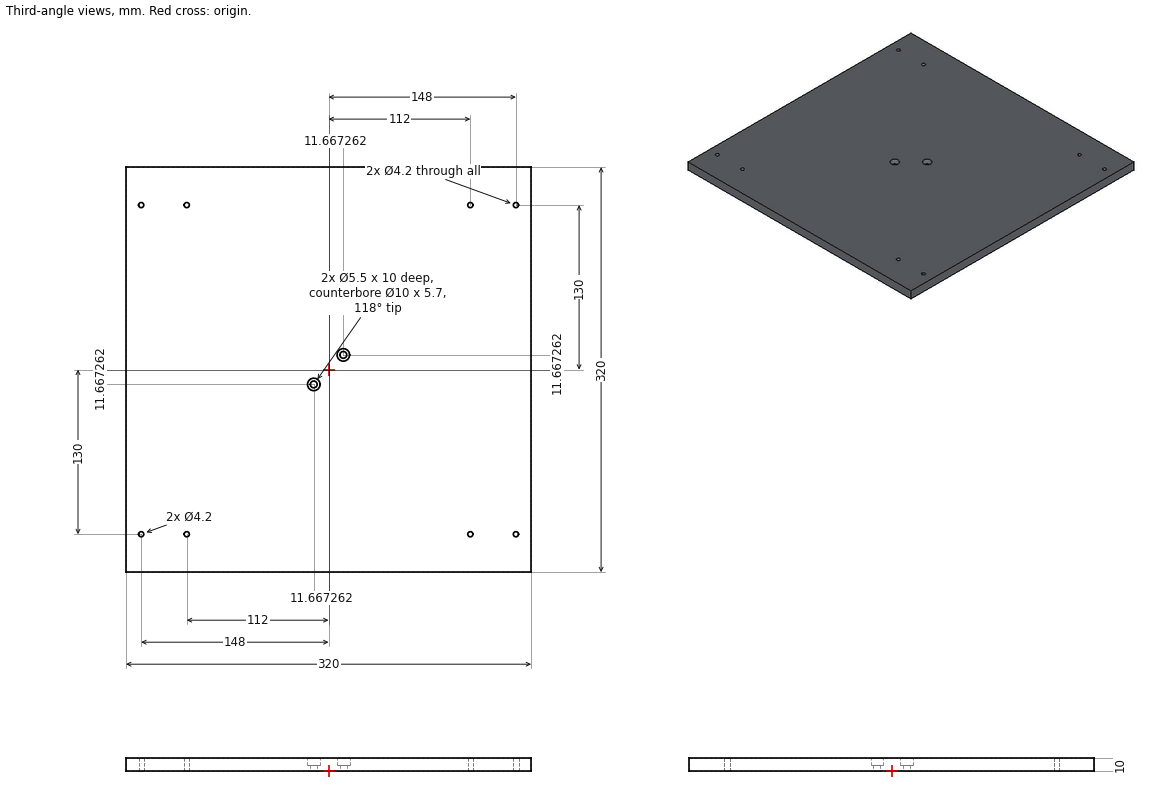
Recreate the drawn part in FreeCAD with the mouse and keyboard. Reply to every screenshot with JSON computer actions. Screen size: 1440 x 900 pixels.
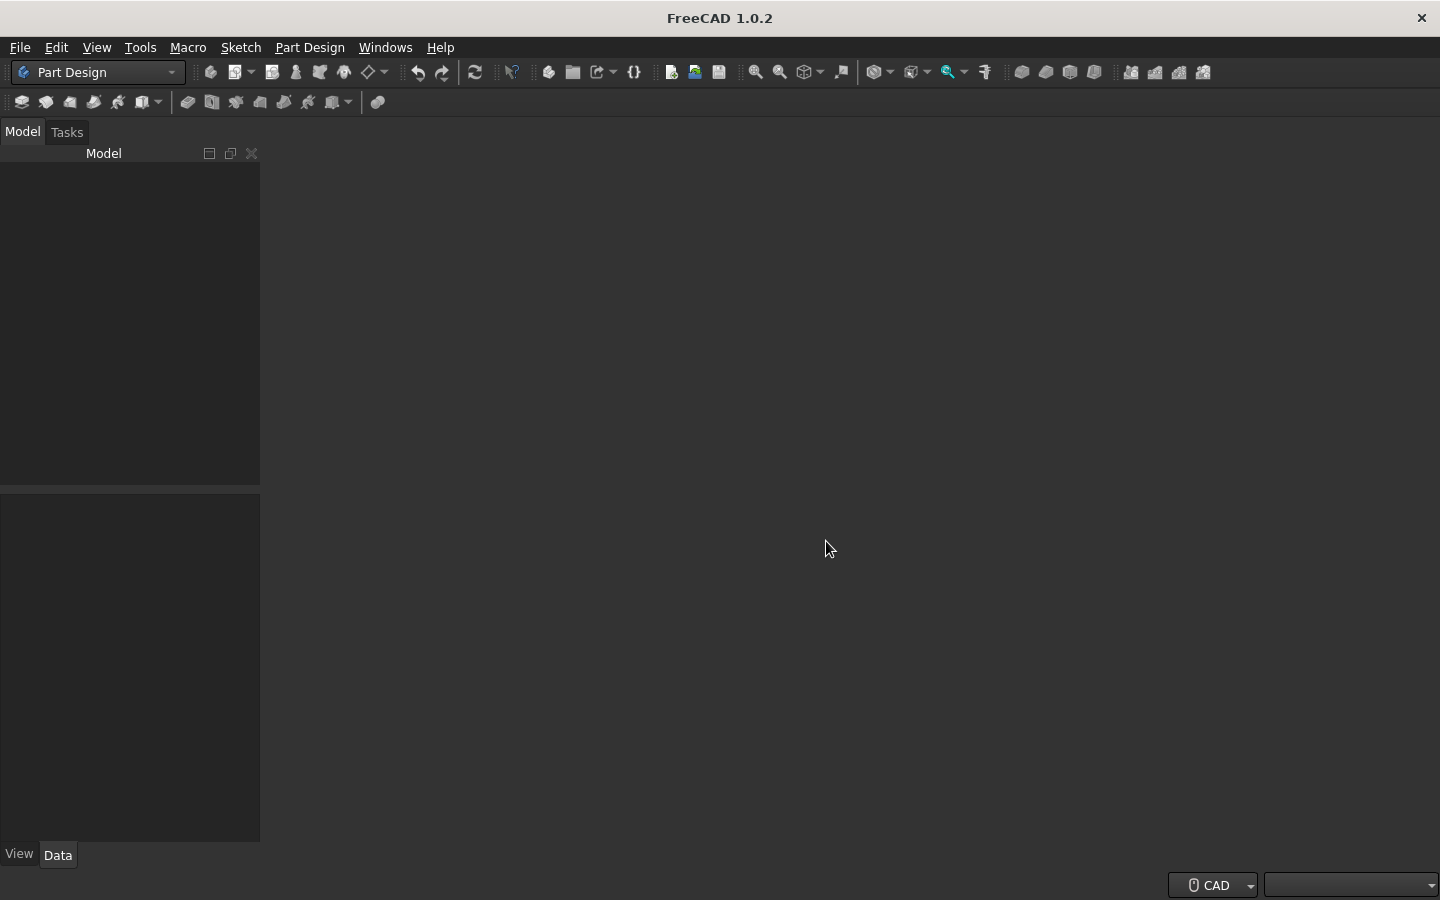
{"action": "key", "text": "ctrl+n"}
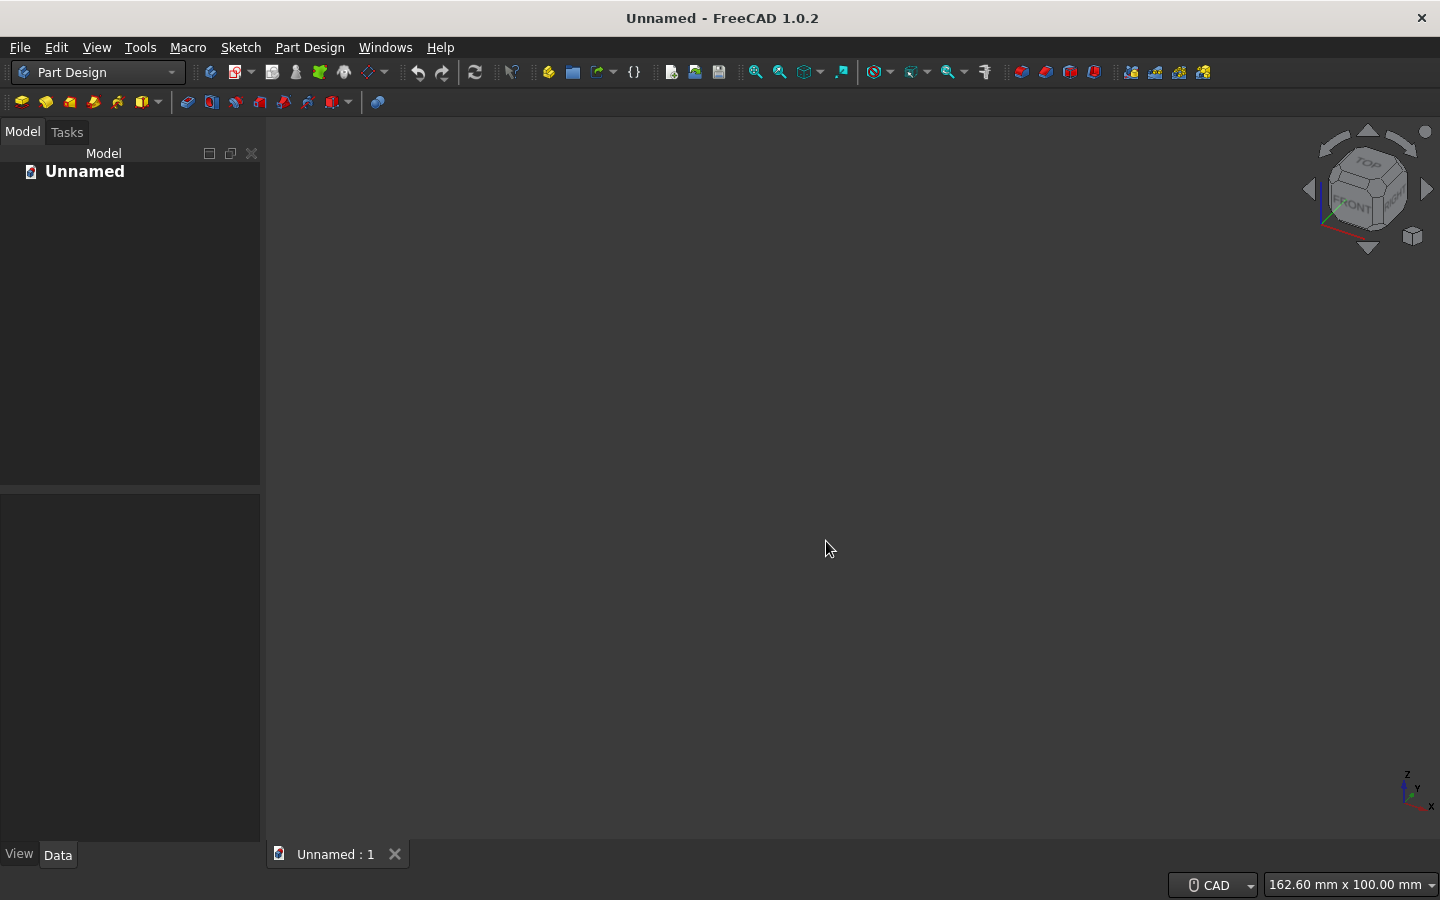
{"action": "left_click", "coordinate": [236, 72]}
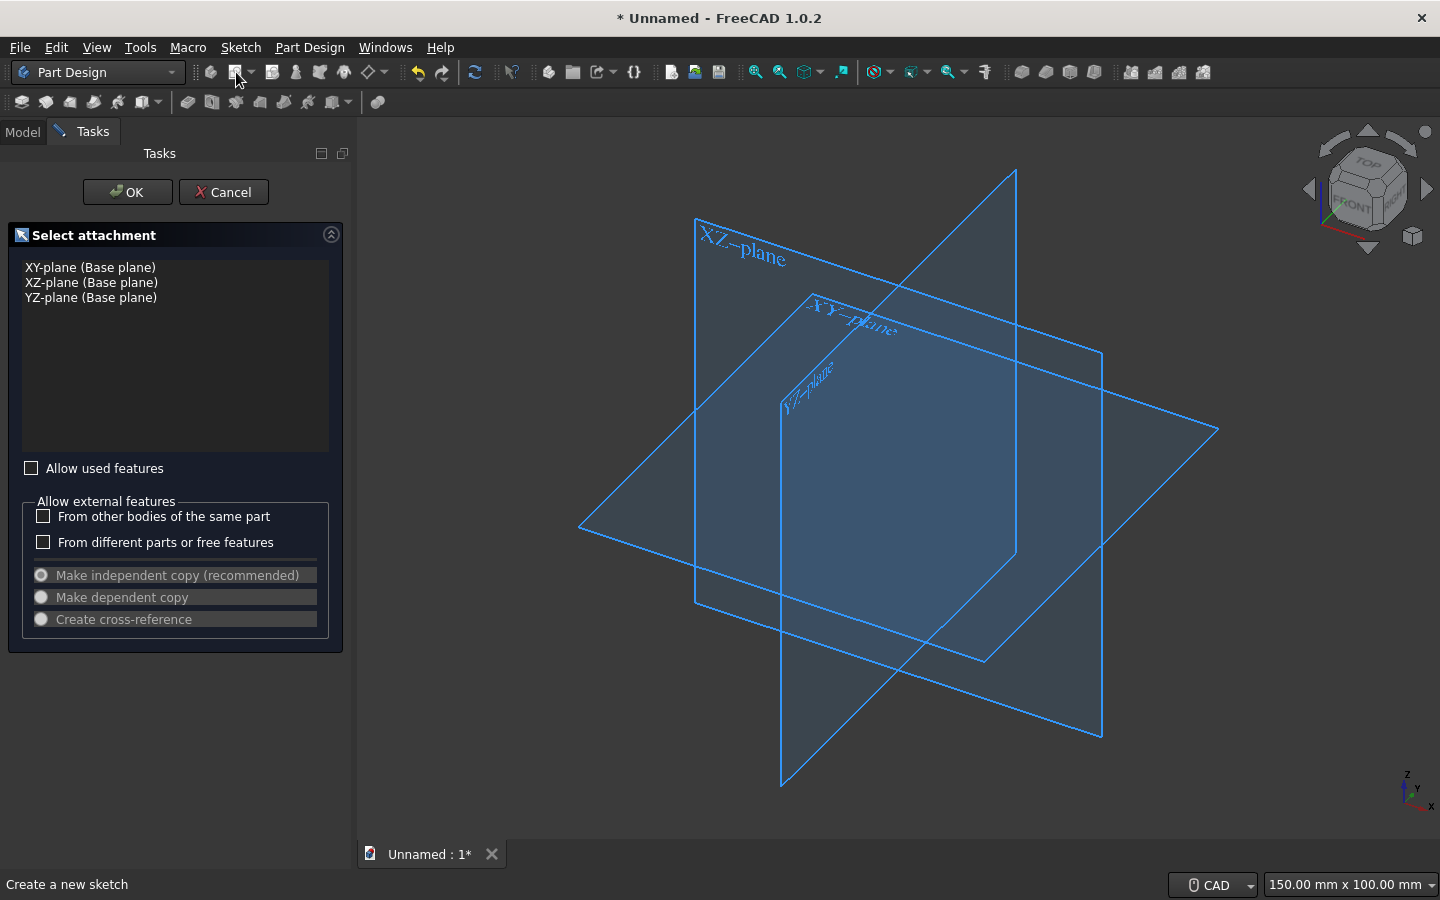
{"action": "left_click", "coordinate": [82, 268]}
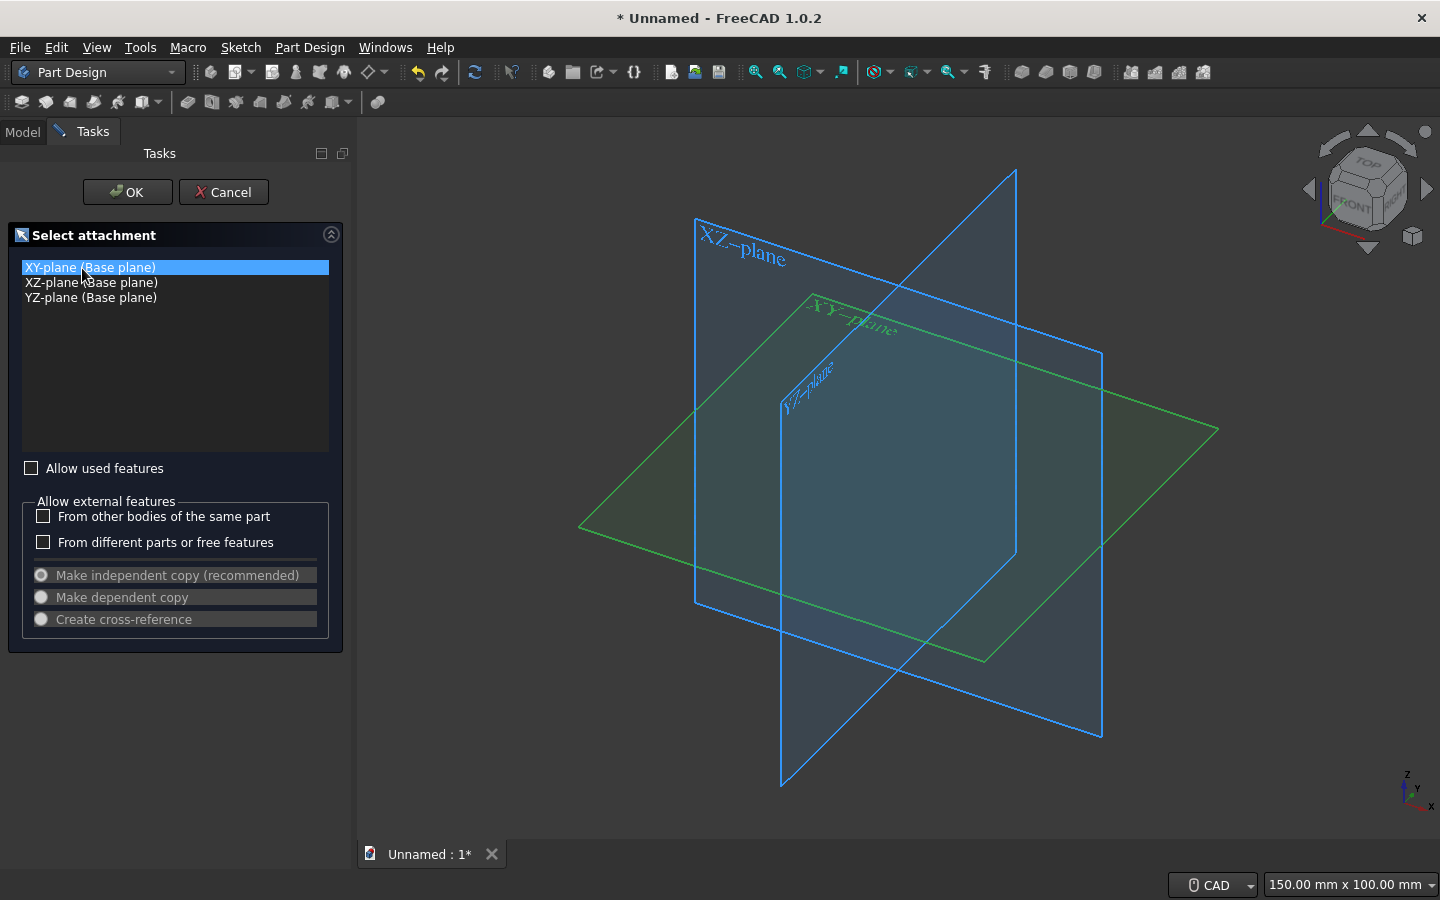
{"action": "left_click", "coordinate": [128, 192]}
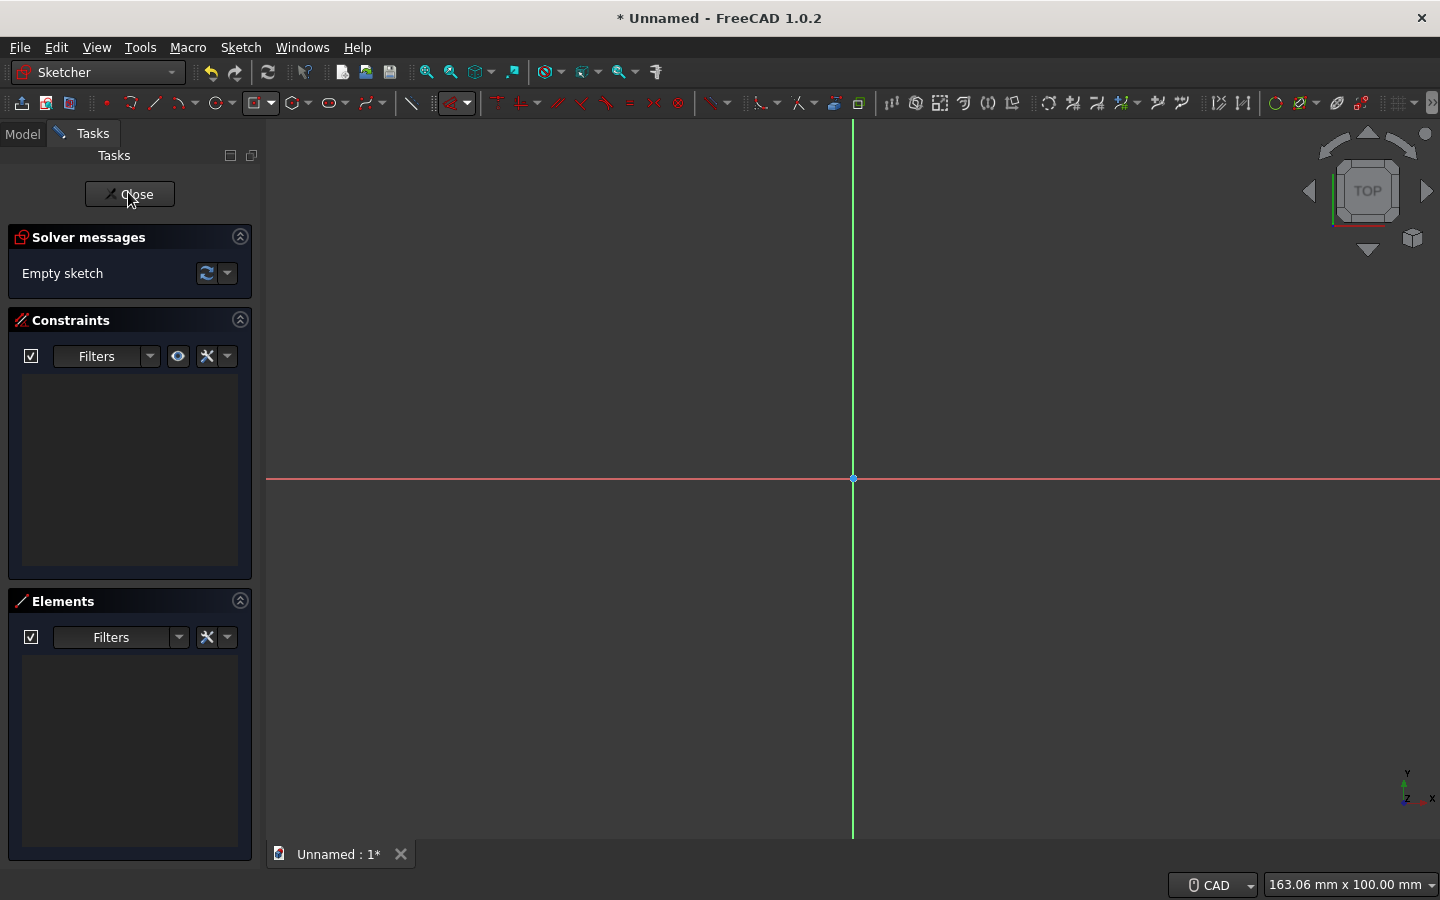
{"action": "scroll", "coordinate": [767, 479], "scroll_direction": "down", "scroll_amount": 8}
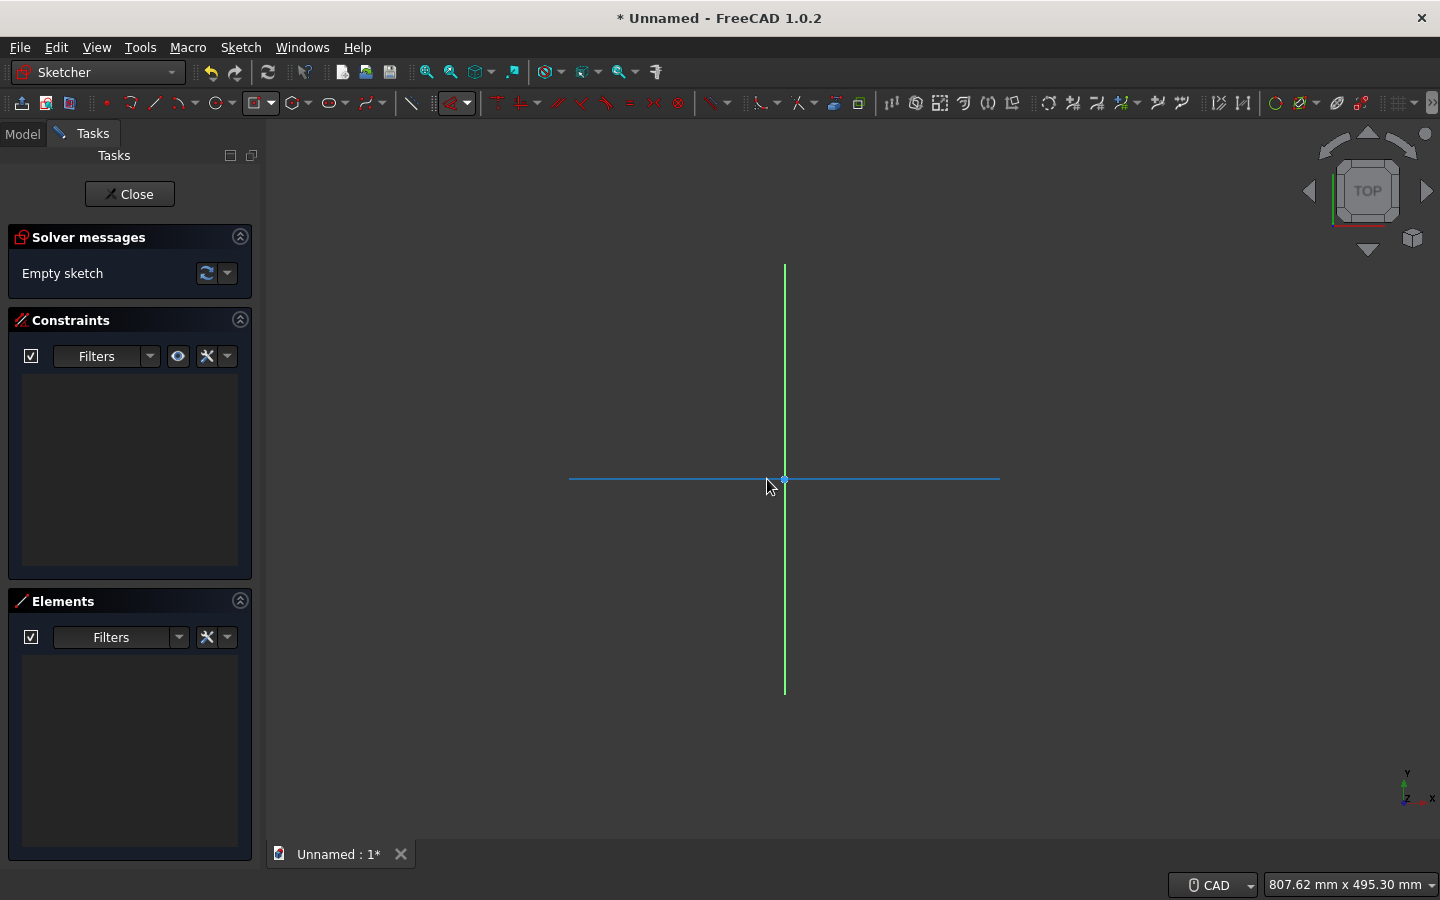
{"action": "left_click", "coordinate": [254, 104]}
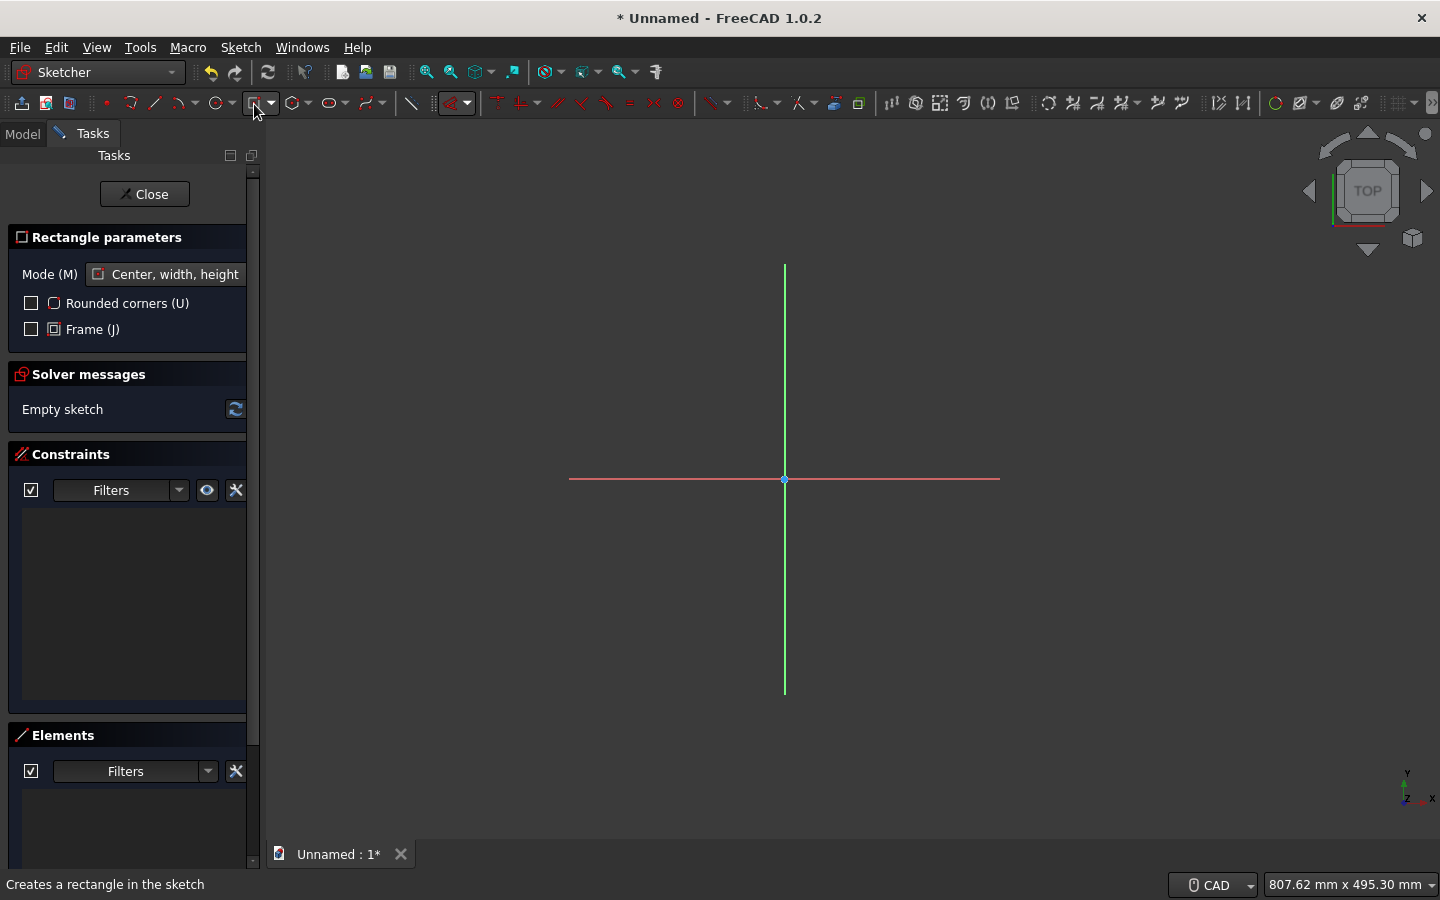
{"action": "left_click", "coordinate": [785, 479]}
{"action": "mouse_move", "coordinate": [1017, 247]}